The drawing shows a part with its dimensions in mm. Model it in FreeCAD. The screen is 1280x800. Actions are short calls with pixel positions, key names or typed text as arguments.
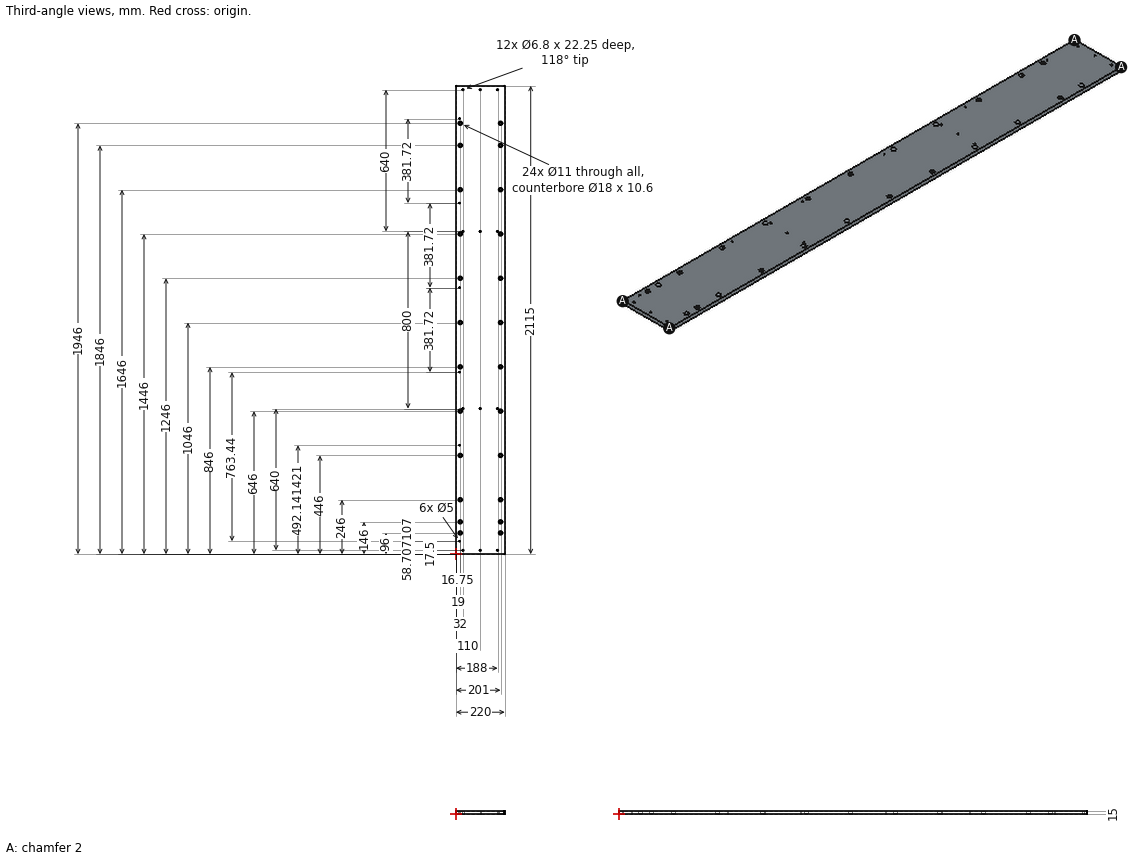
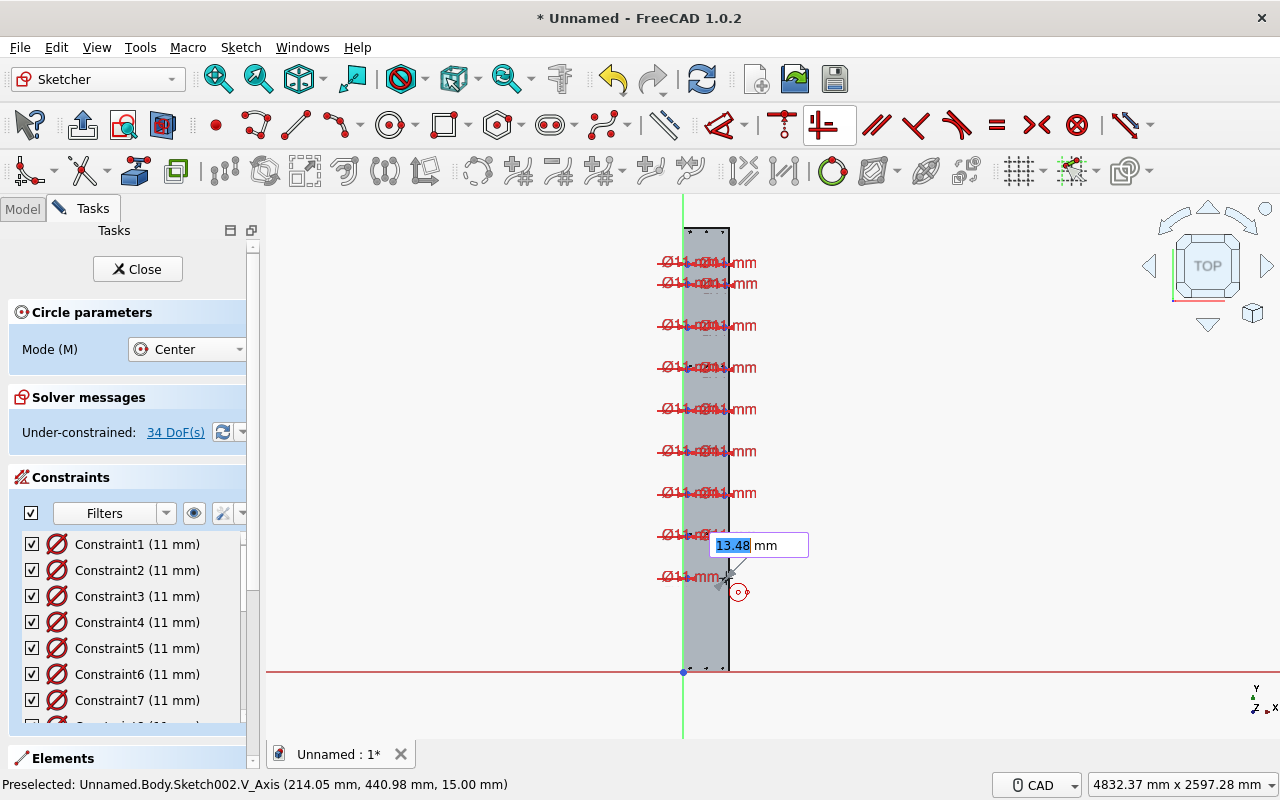
text(11)
key(Return)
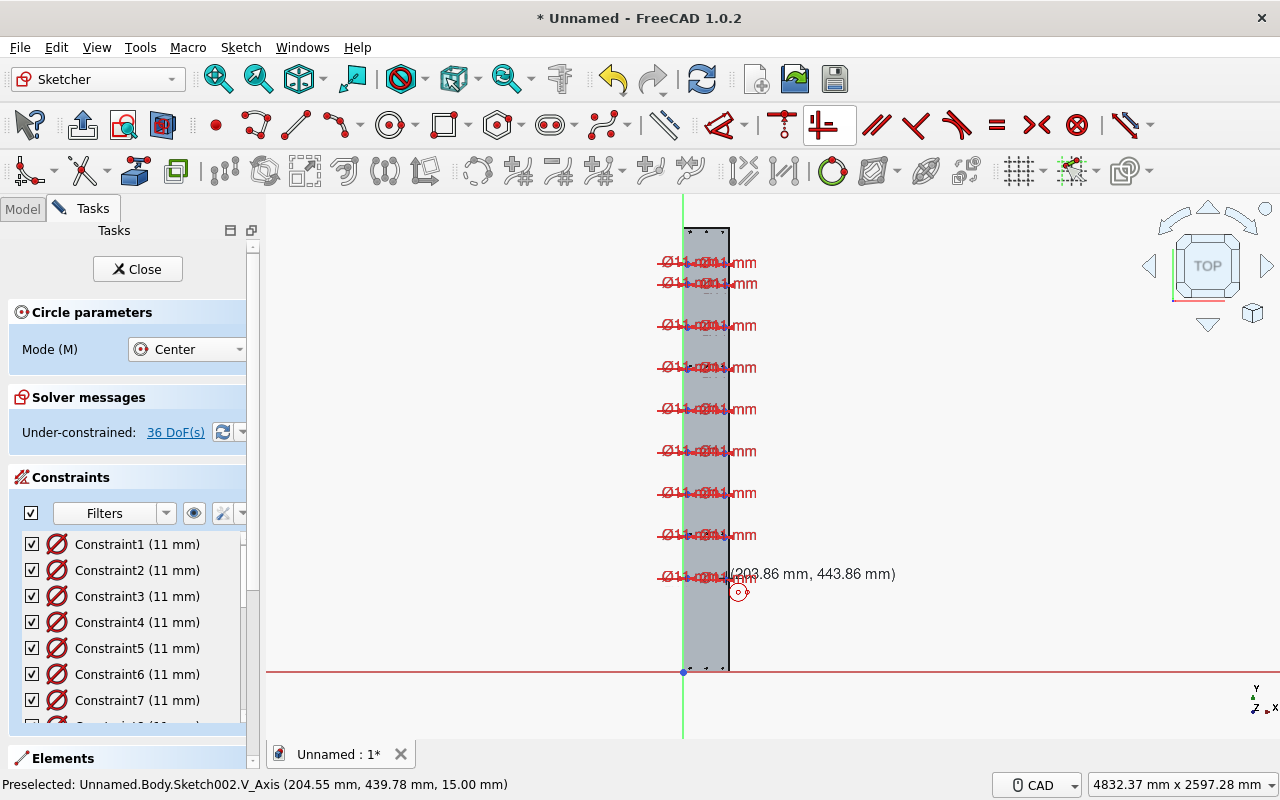
scroll(687, 621, up, 15)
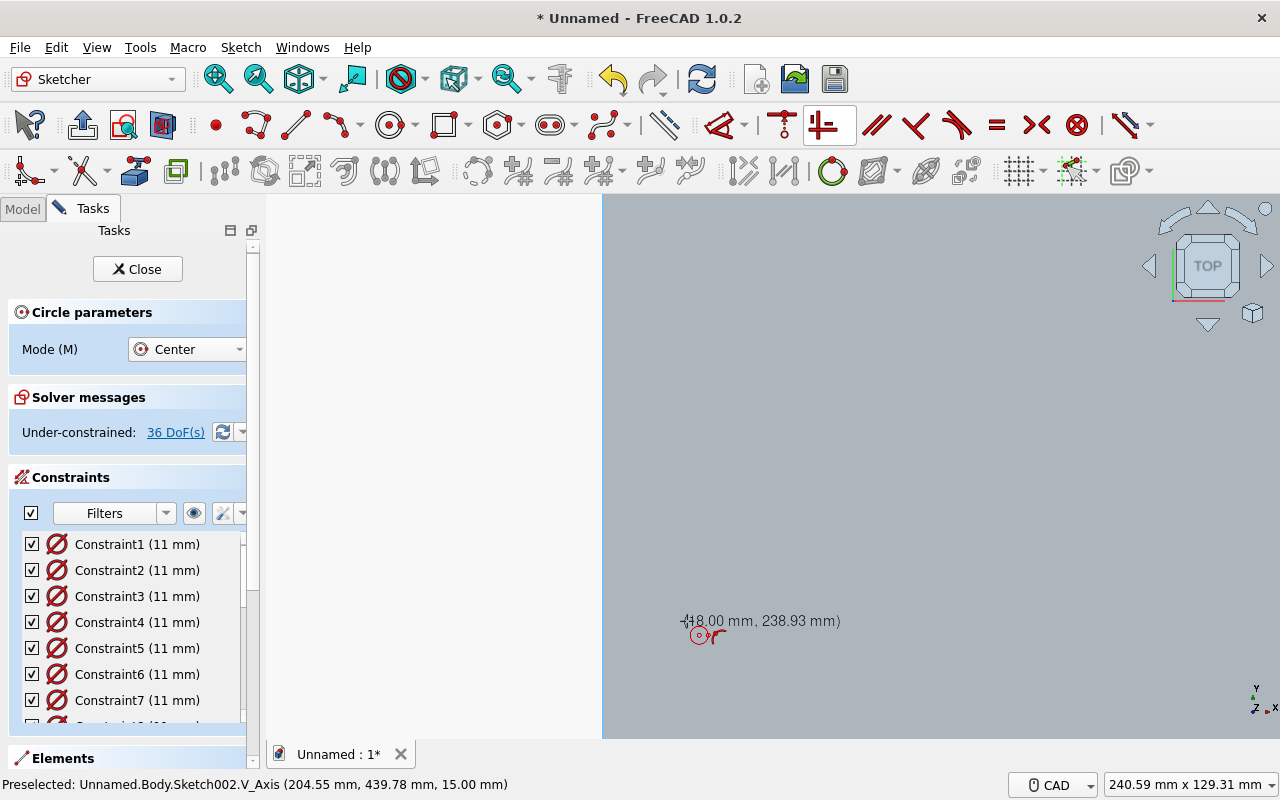
scroll(687, 621, down, 15)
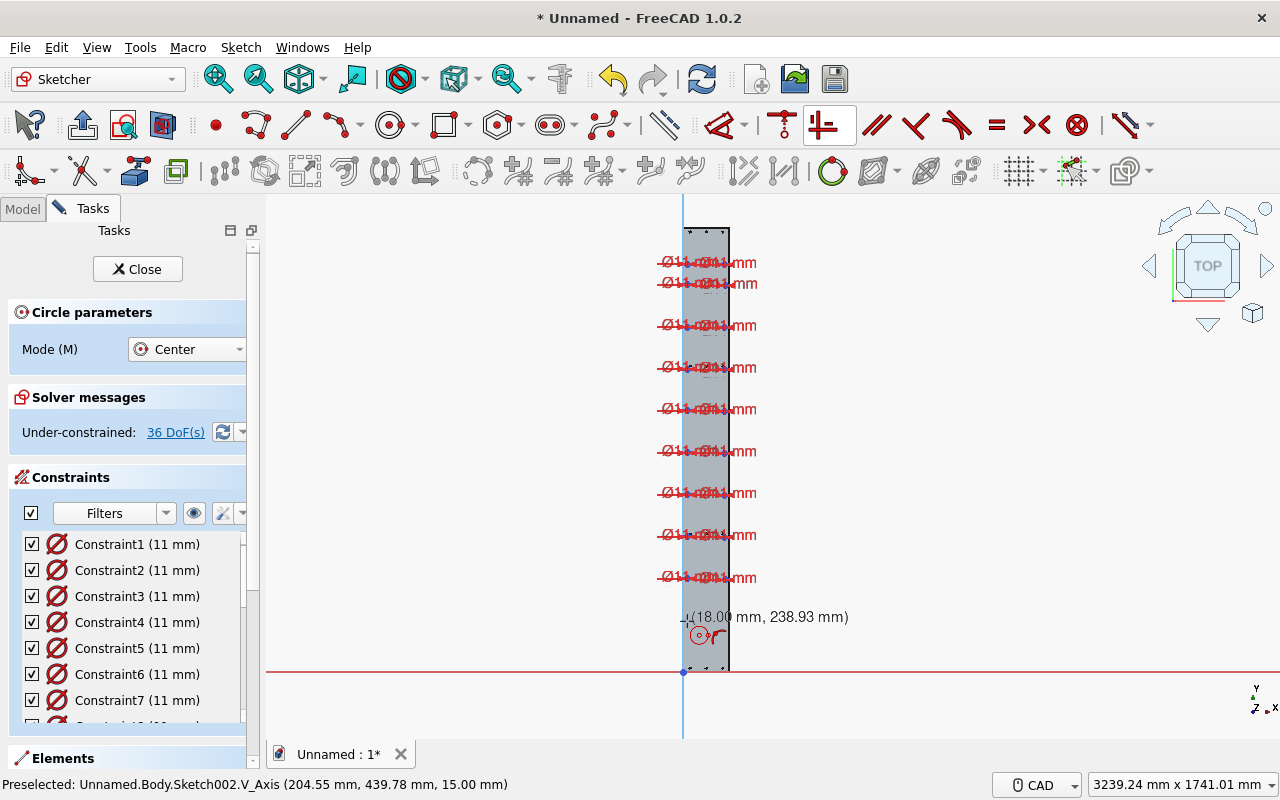
scroll(687, 621, up, 7)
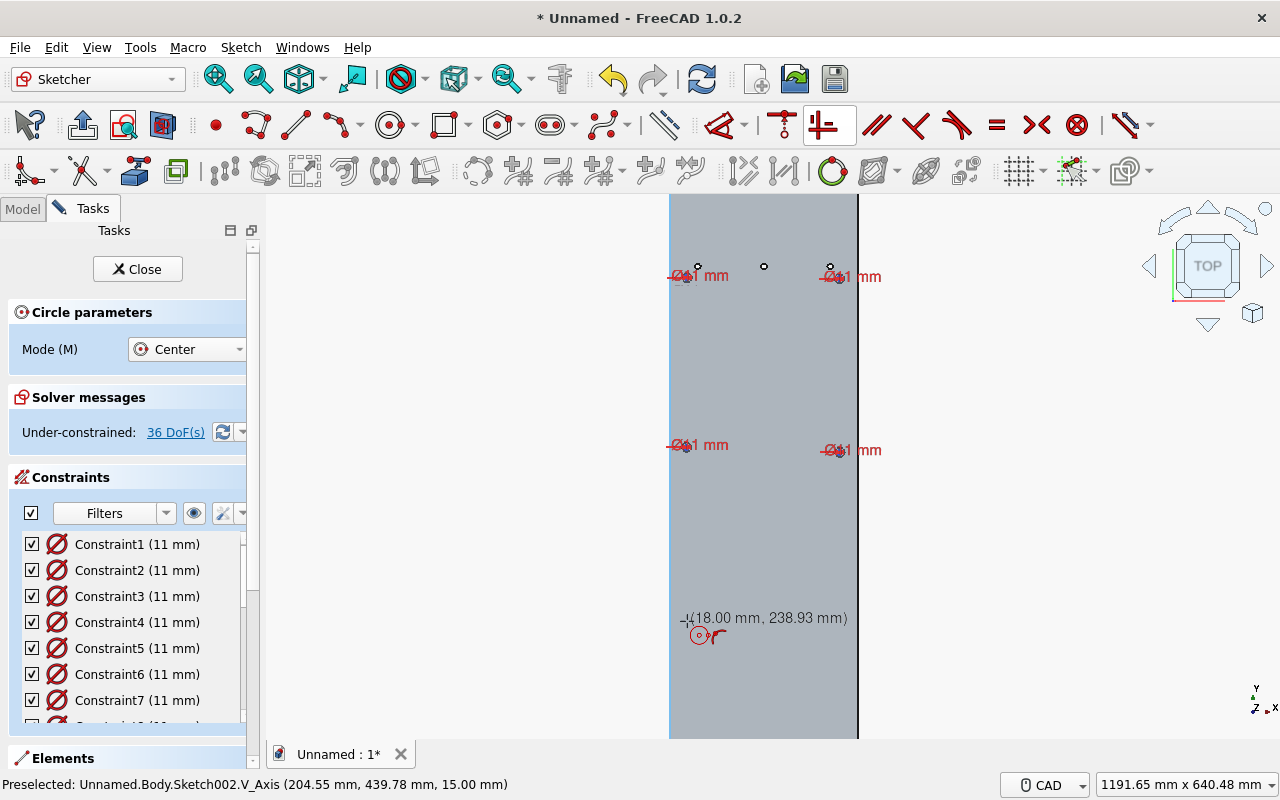
click(687, 617)
move(690, 613)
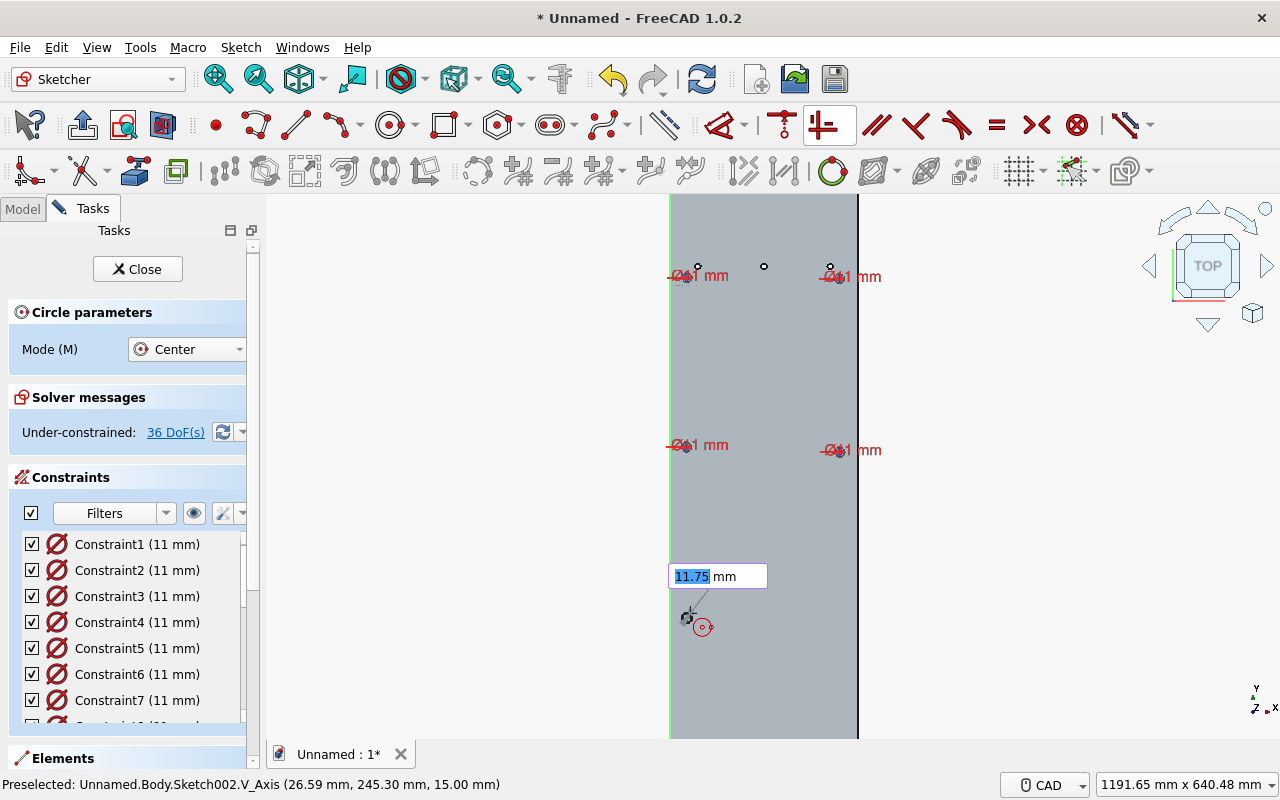
text(11)
key(Return)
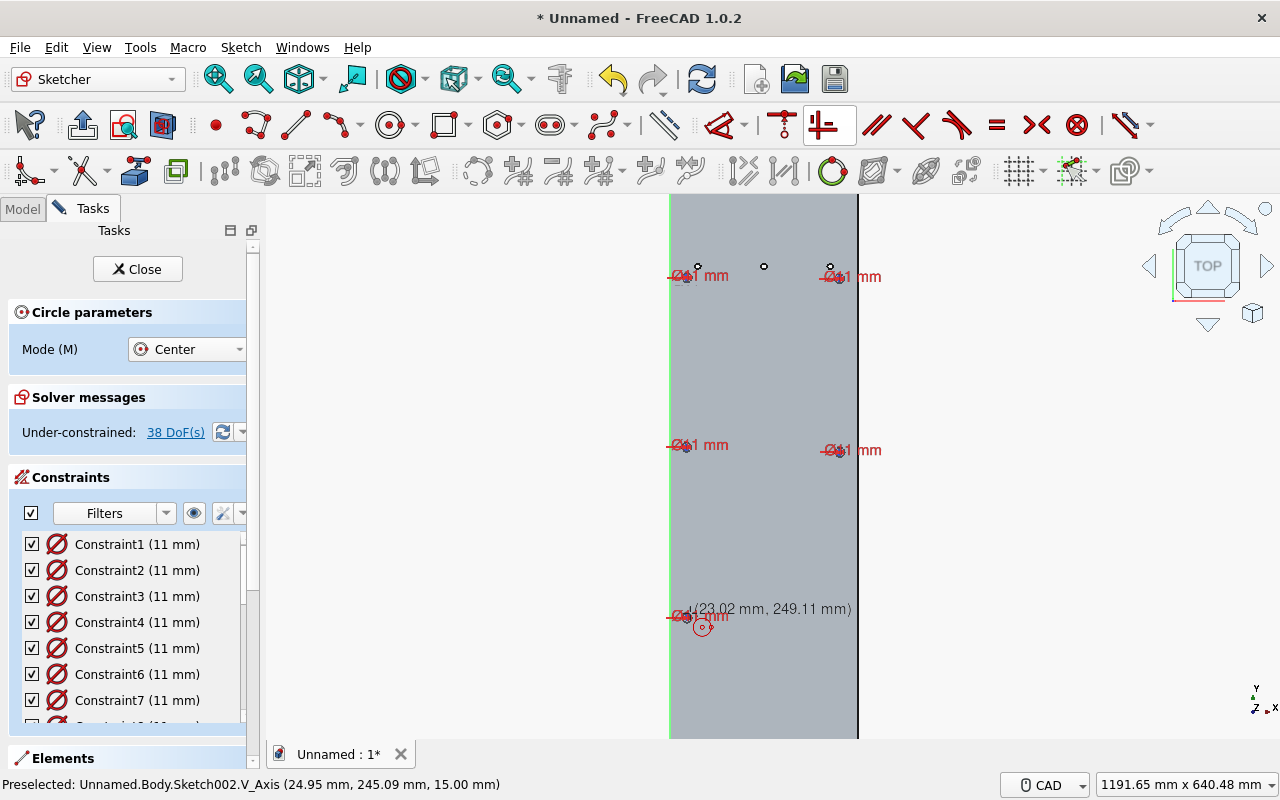
scroll(841, 617, up, 8)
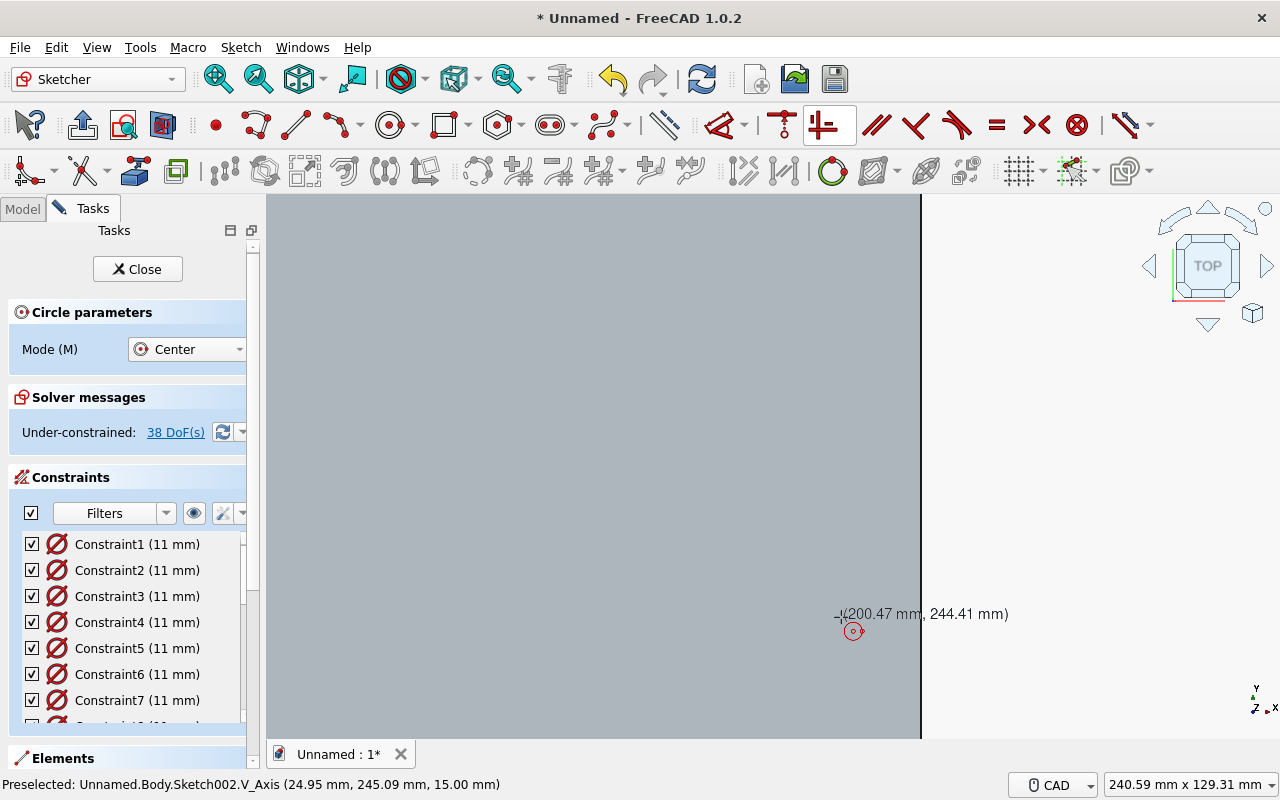
scroll(719, 620, down, 15)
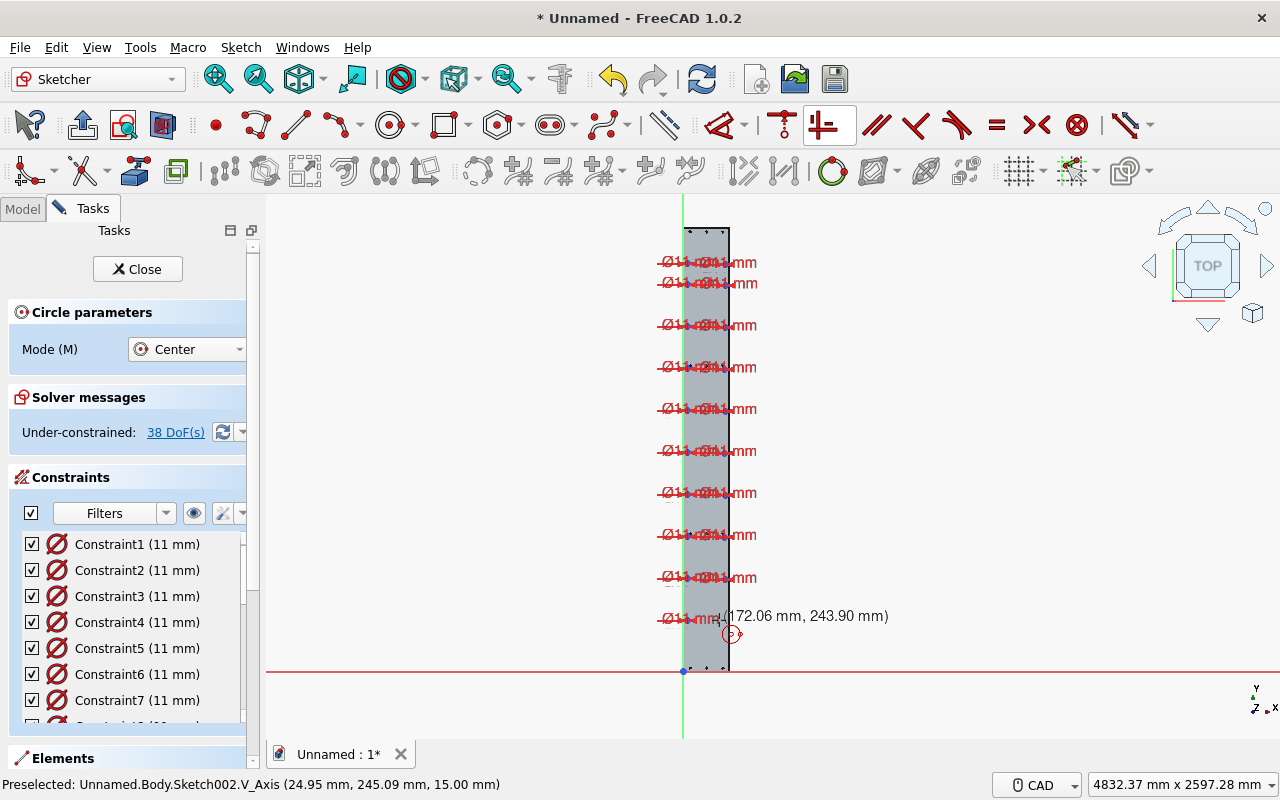
click(725, 620)
move(726, 620)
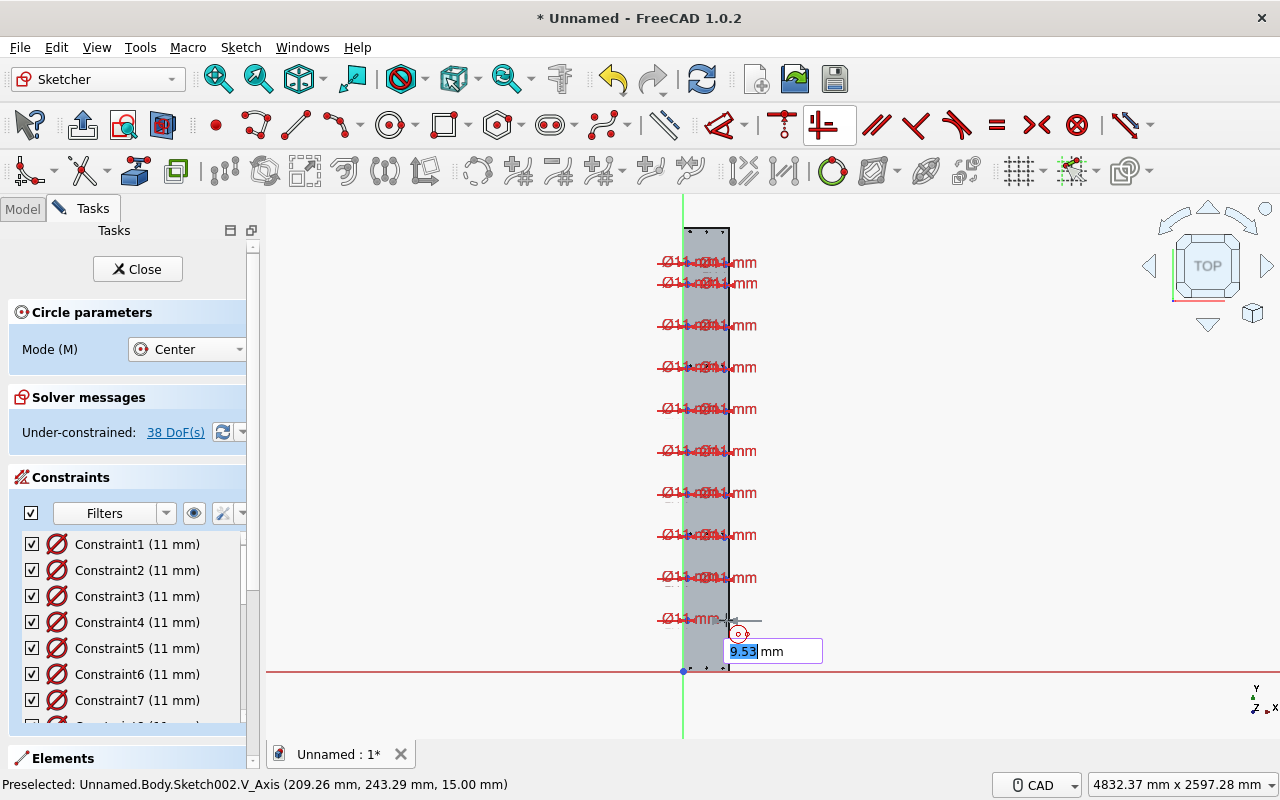
text(11)
key(Return)